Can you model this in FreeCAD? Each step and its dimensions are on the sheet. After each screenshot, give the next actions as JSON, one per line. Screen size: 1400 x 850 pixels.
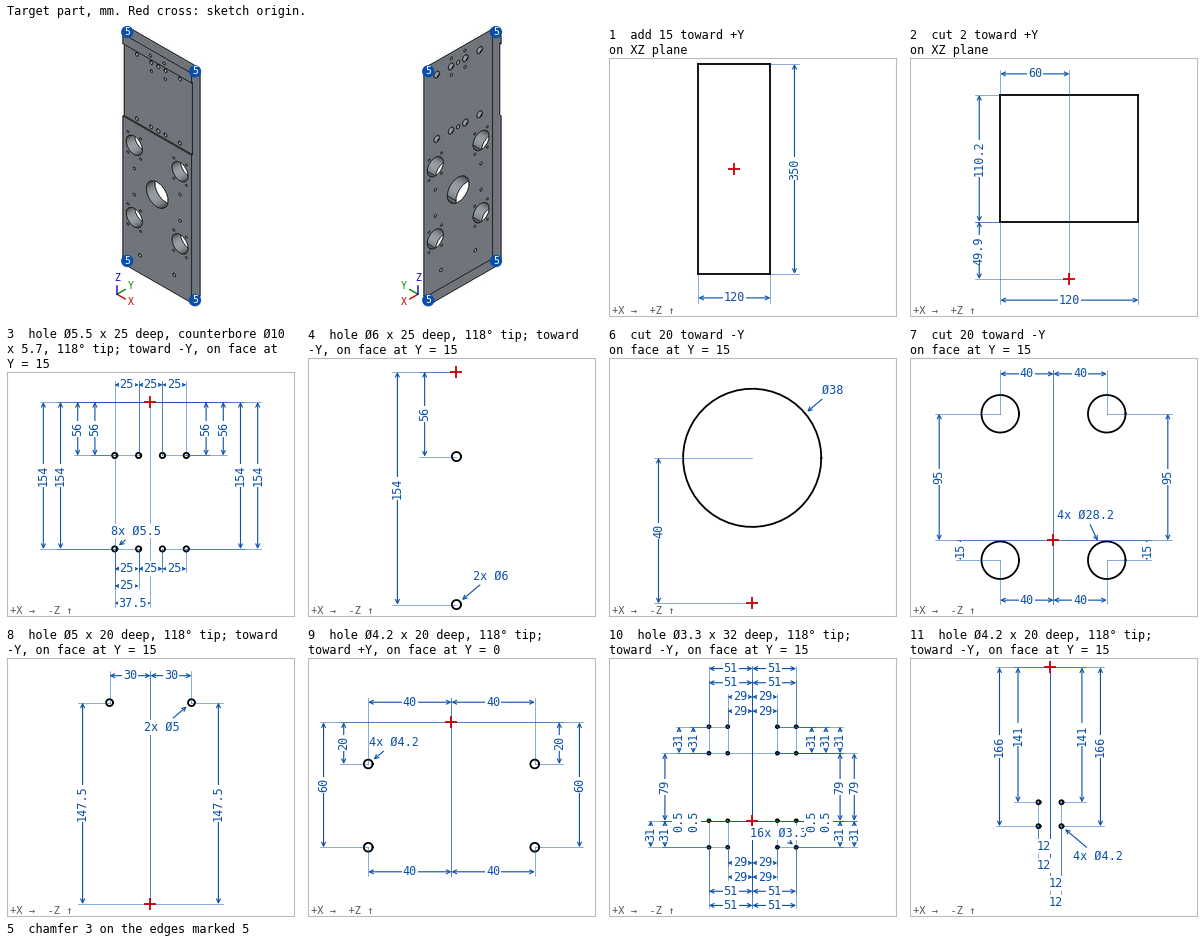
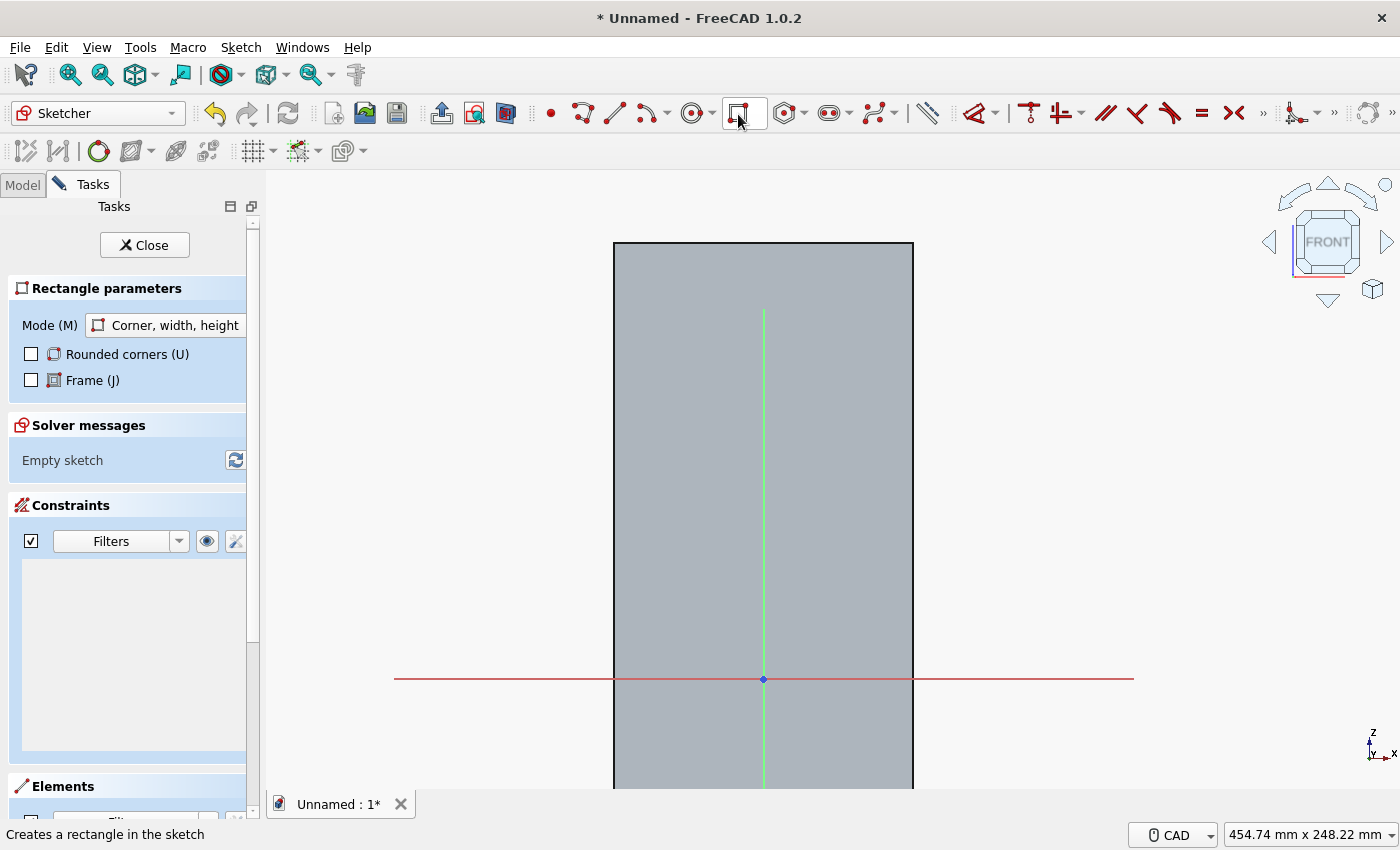
{"action": "left_click", "coordinate": [614, 280]}
{"action": "left_click", "coordinate": [913, 555]}
{"action": "key", "text": "Escape"}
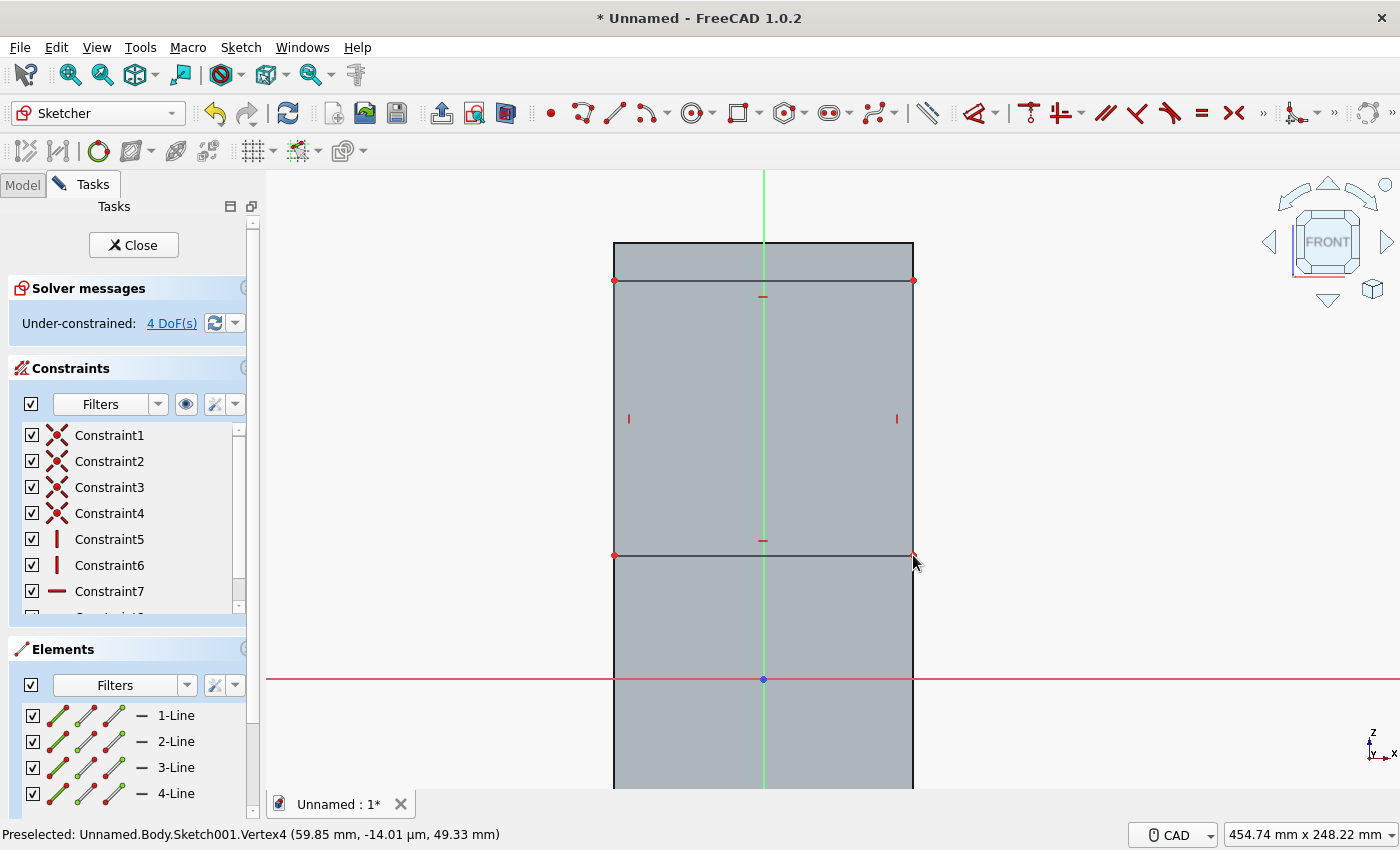
{"action": "left_click", "coordinate": [974, 114]}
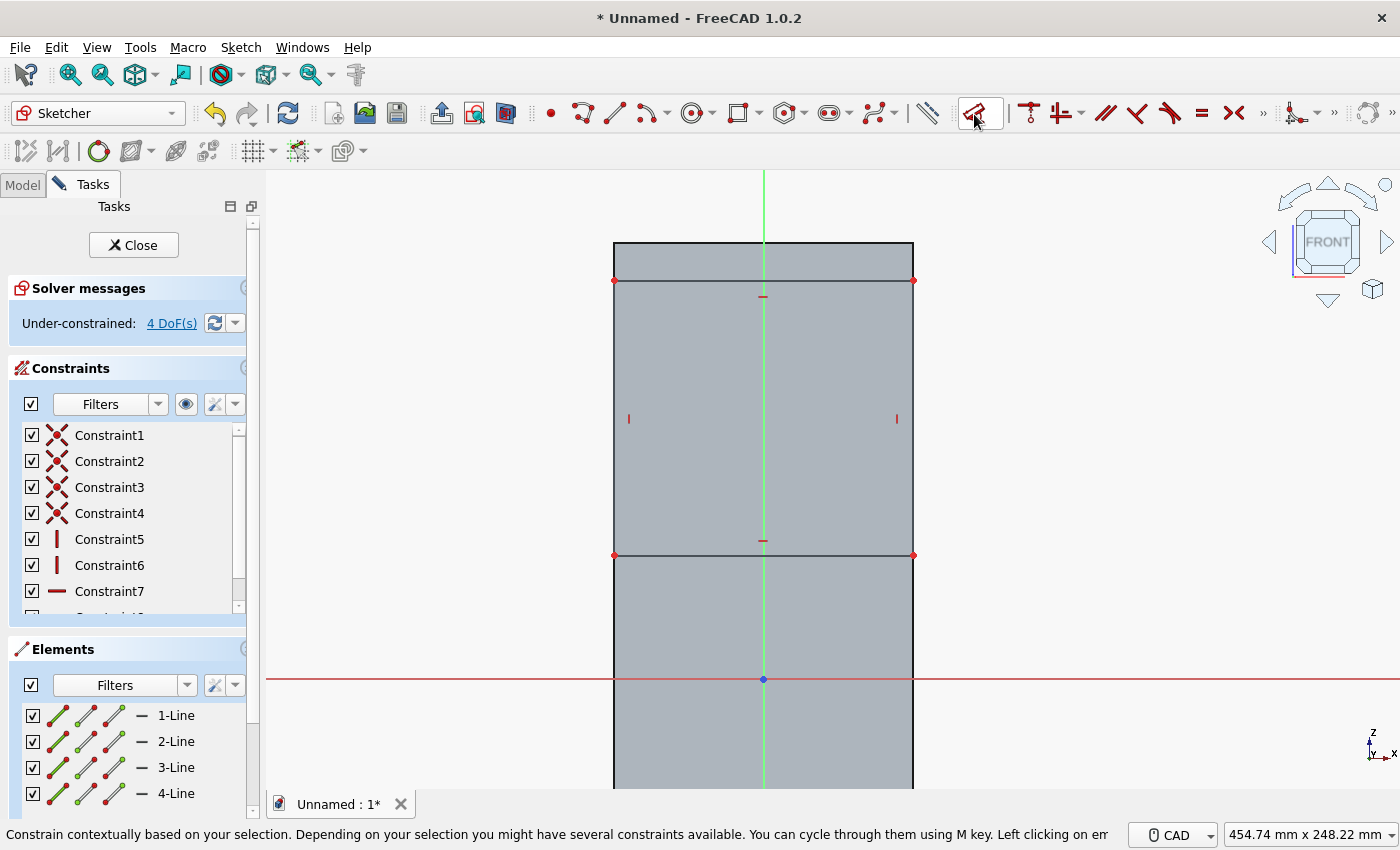
{"action": "left_click", "coordinate": [704, 556]}
{"action": "left_click", "coordinate": [695, 590]}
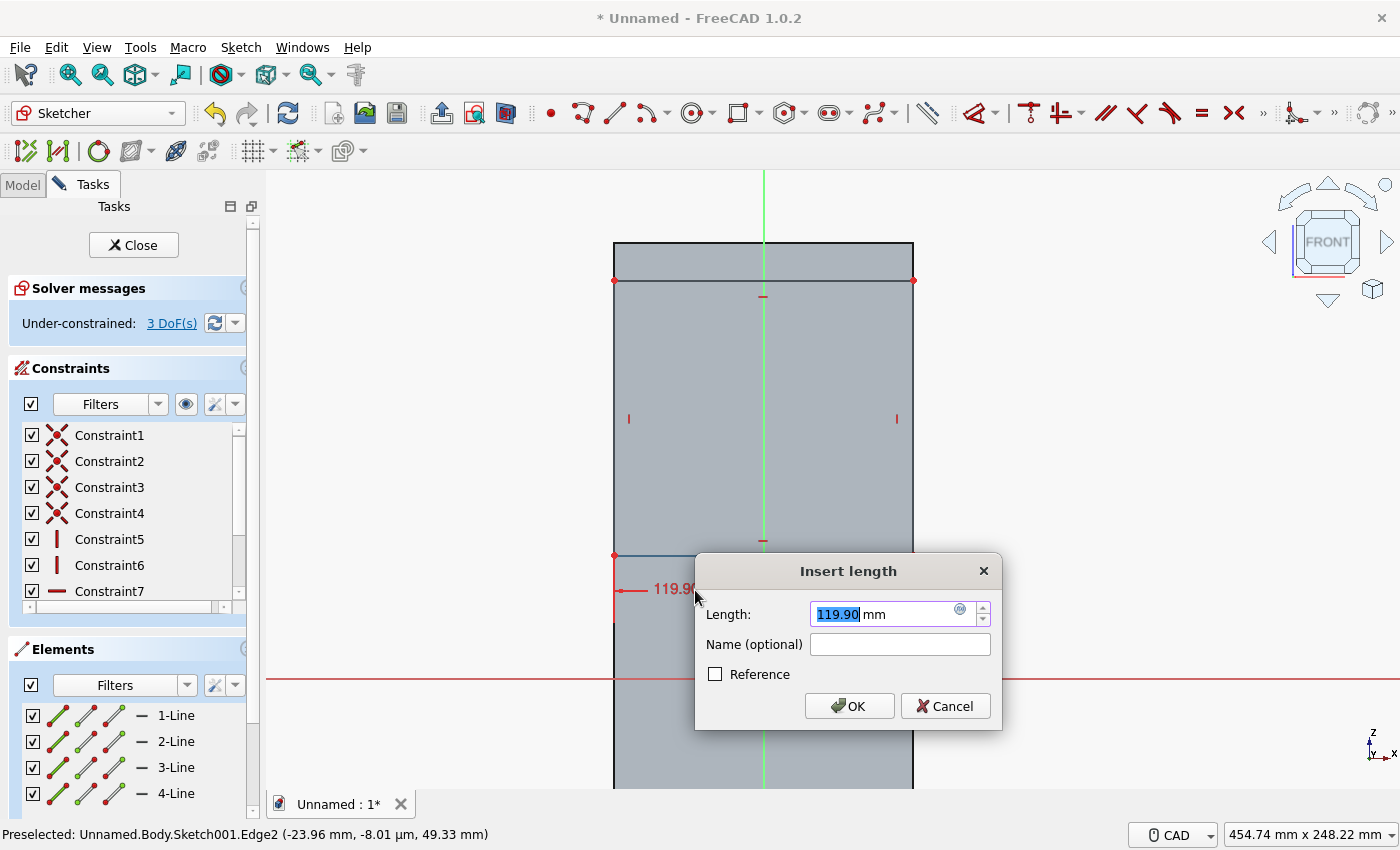
{"action": "type", "text": "120"}
{"action": "key", "text": "Return"}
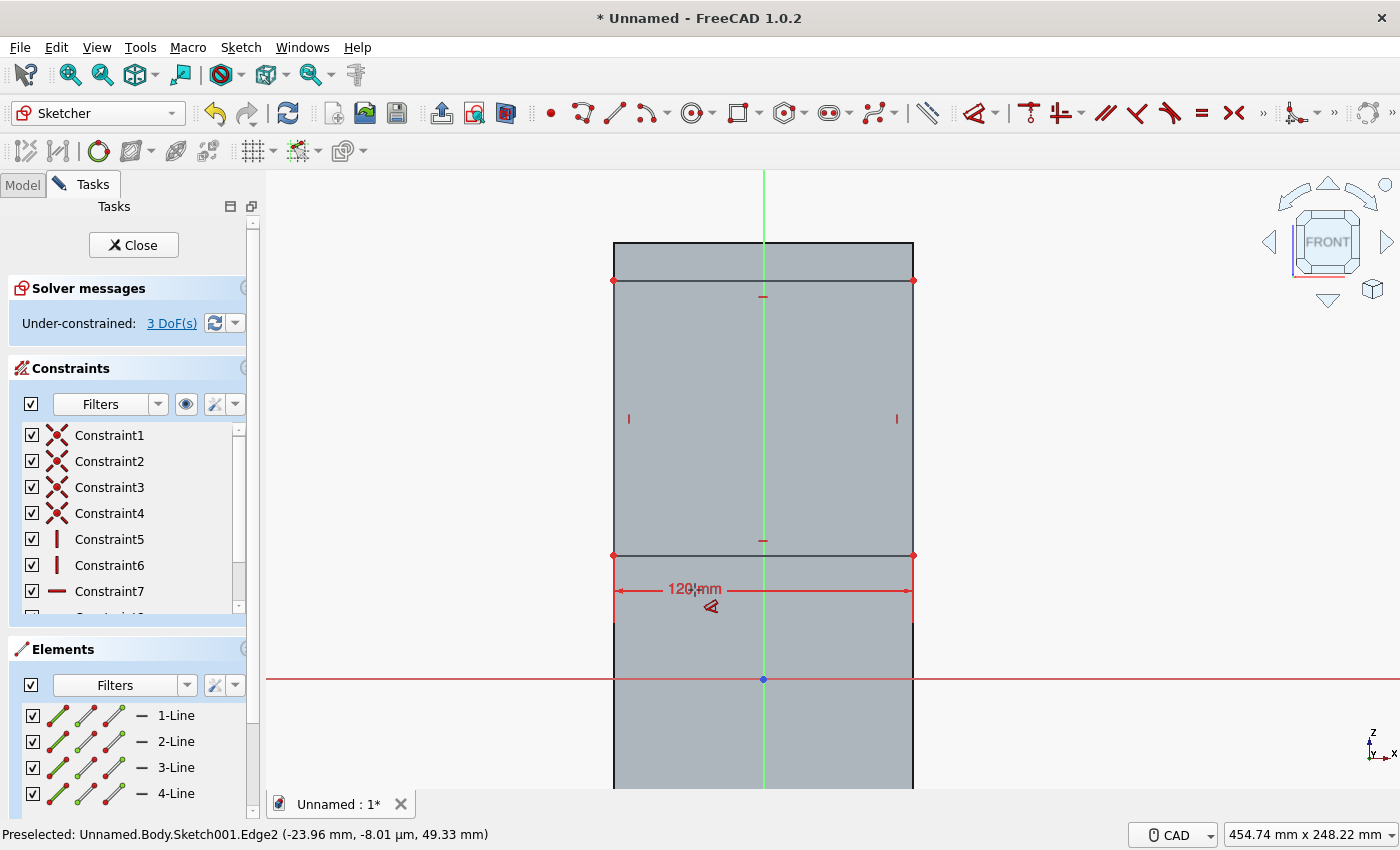
{"action": "left_click", "coordinate": [614, 281]}
{"action": "left_click", "coordinate": [689, 713]}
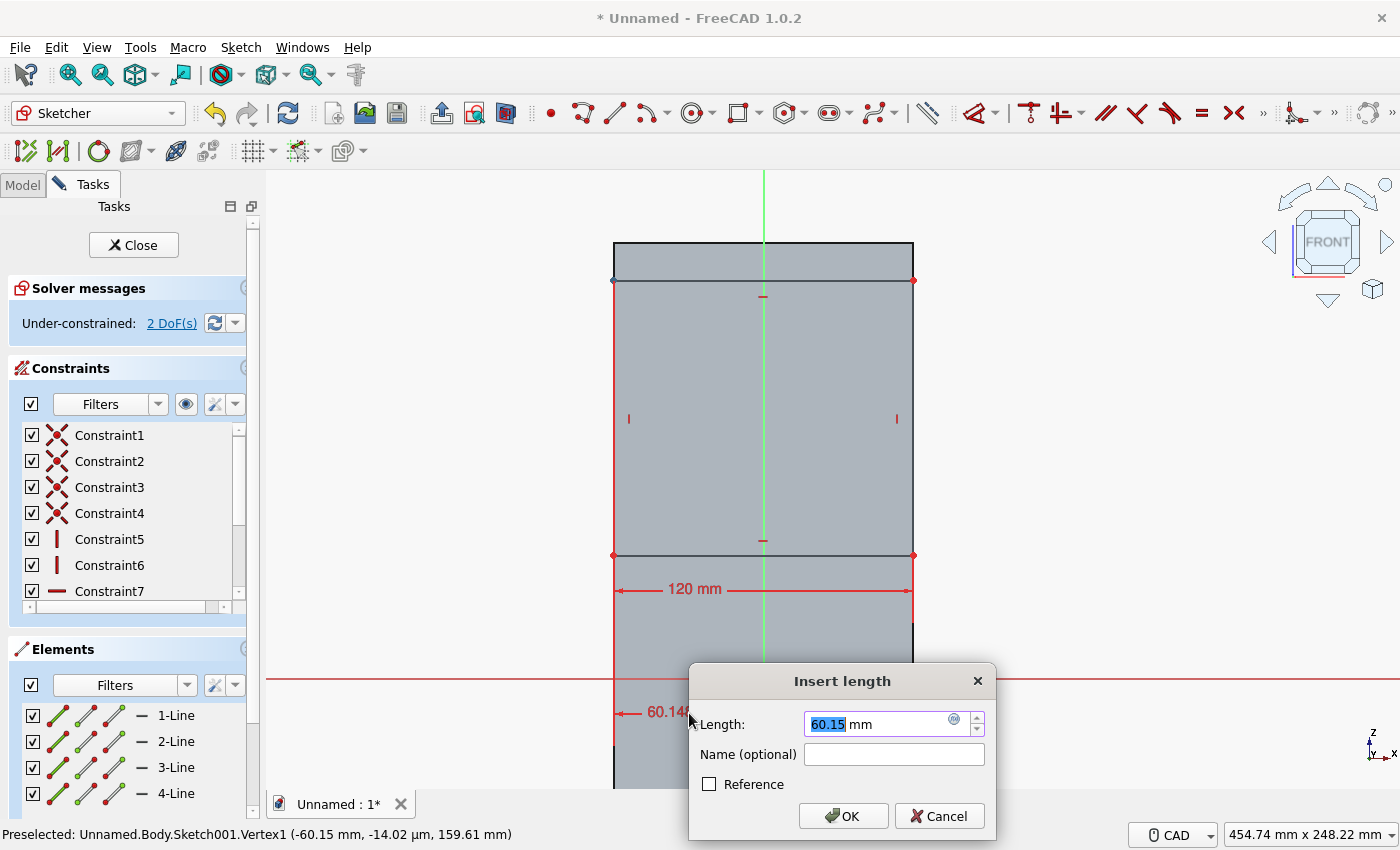
{"action": "type", "text": "60"}
{"action": "key", "text": "Return"}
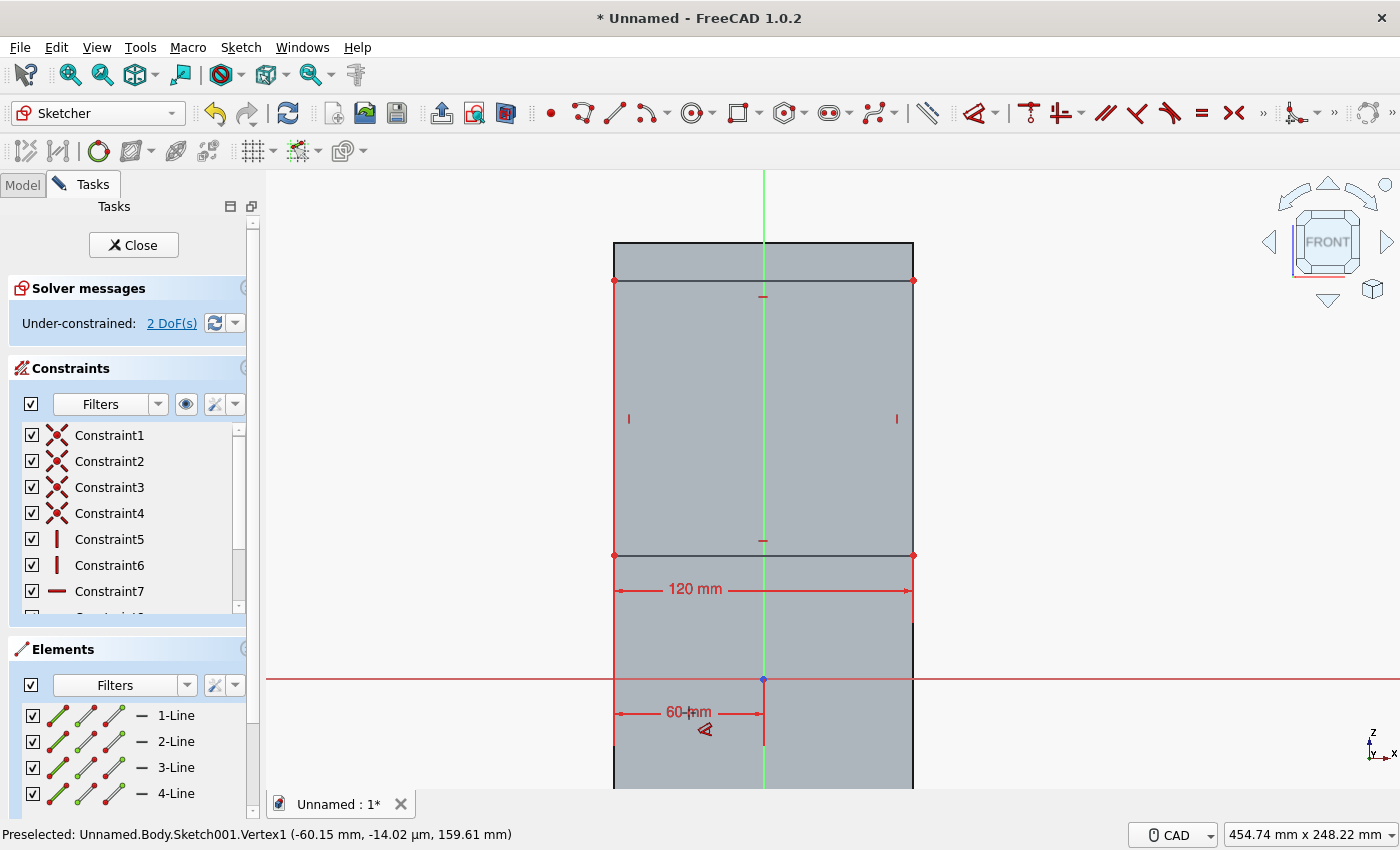
{"action": "left_click", "coordinate": [614, 364]}
{"action": "left_click", "coordinate": [580, 419]}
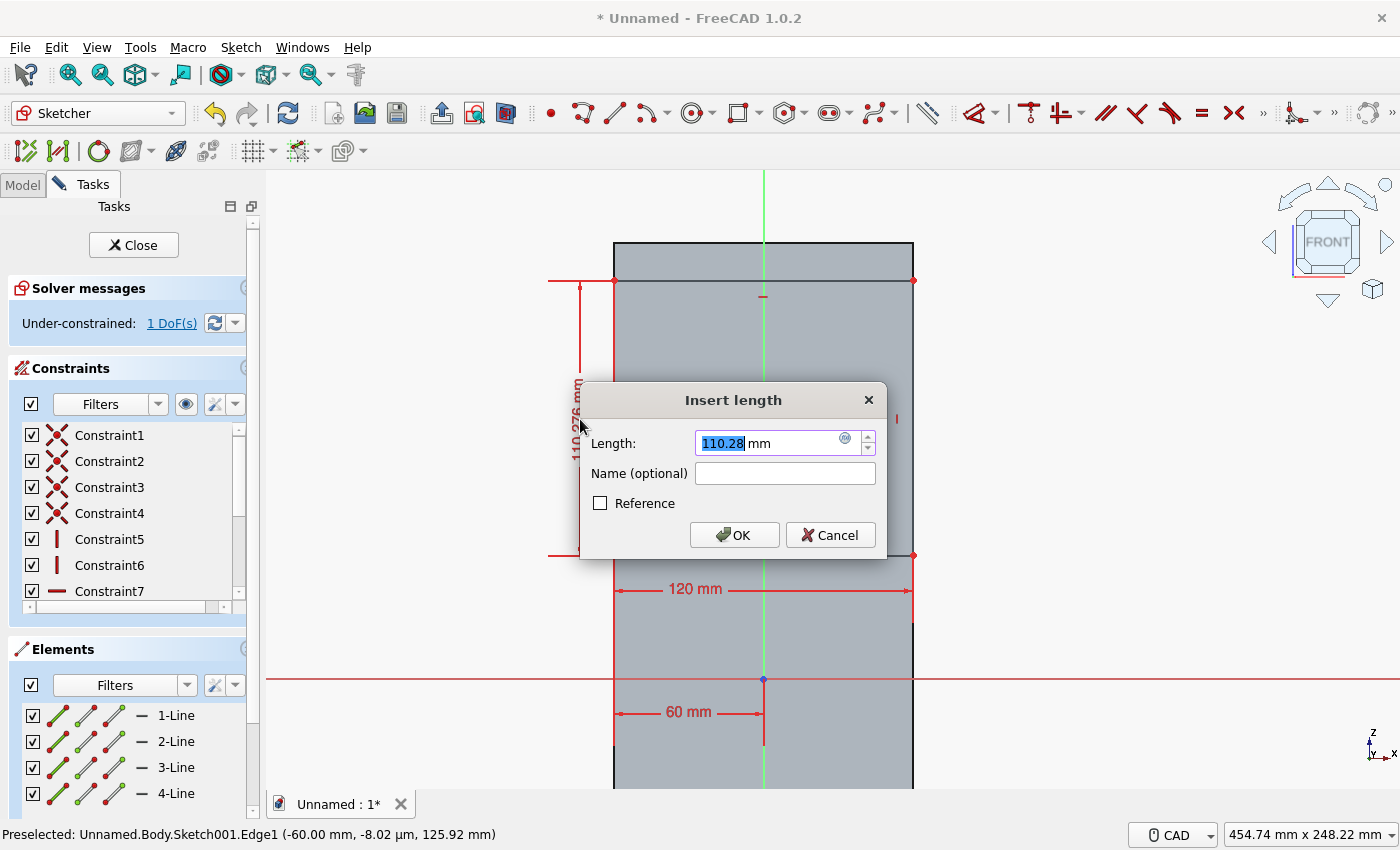
{"action": "type", "text": "110.2"}
{"action": "key", "text": "Return"}